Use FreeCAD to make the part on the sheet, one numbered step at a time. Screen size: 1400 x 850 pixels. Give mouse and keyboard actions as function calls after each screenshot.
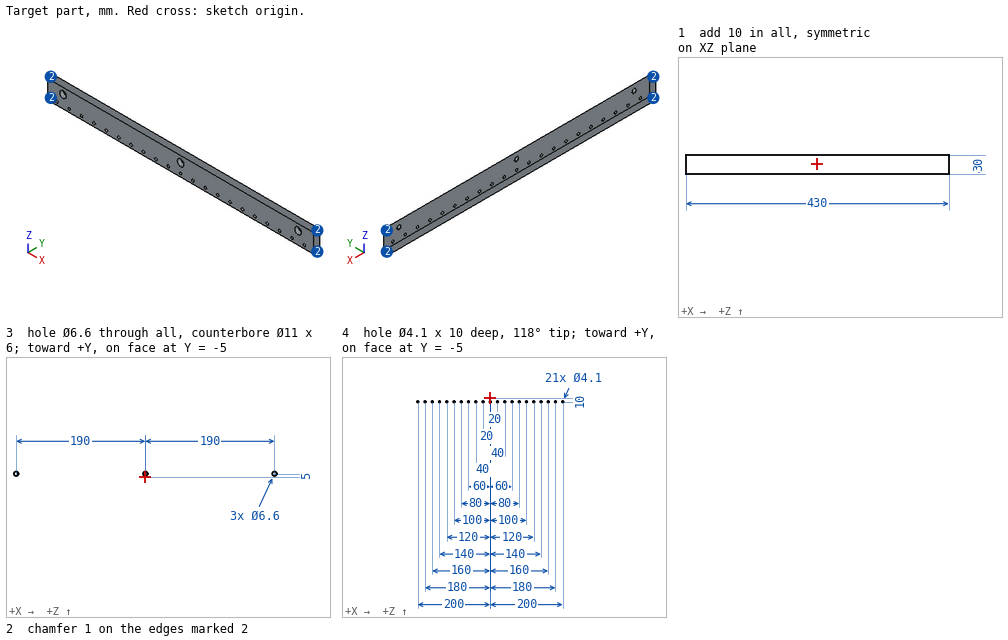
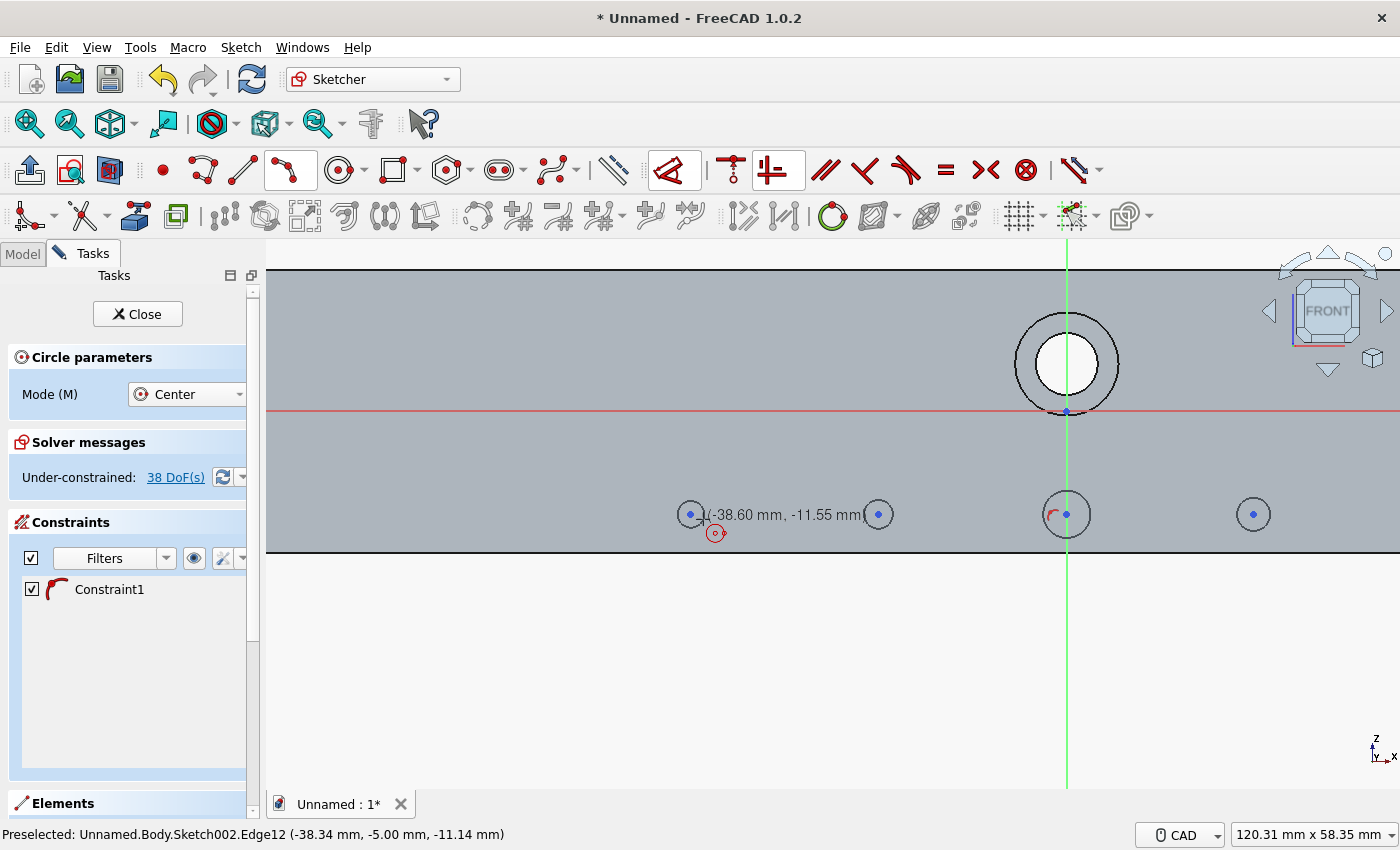
scroll(705, 523, down, 9)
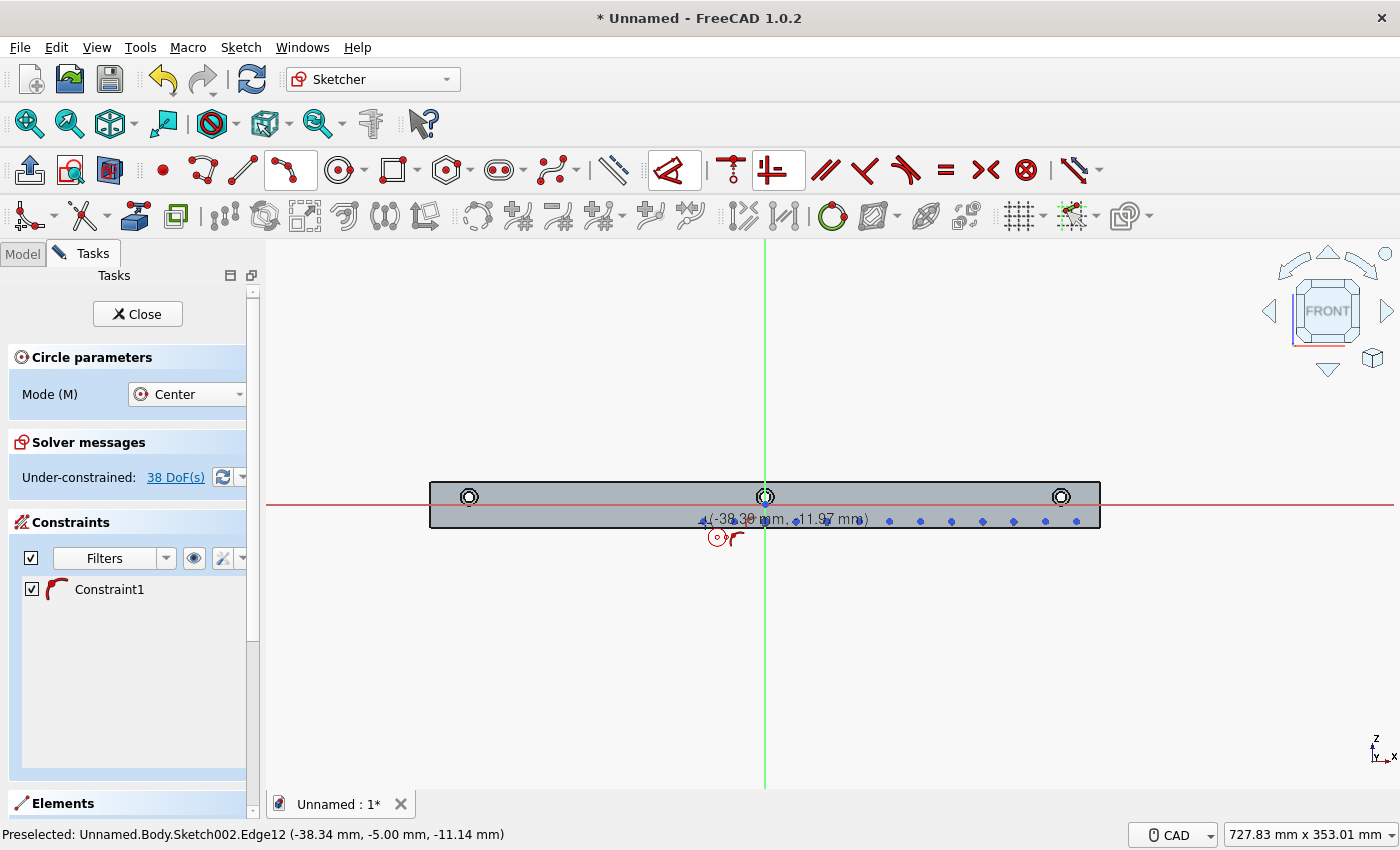
click(672, 521)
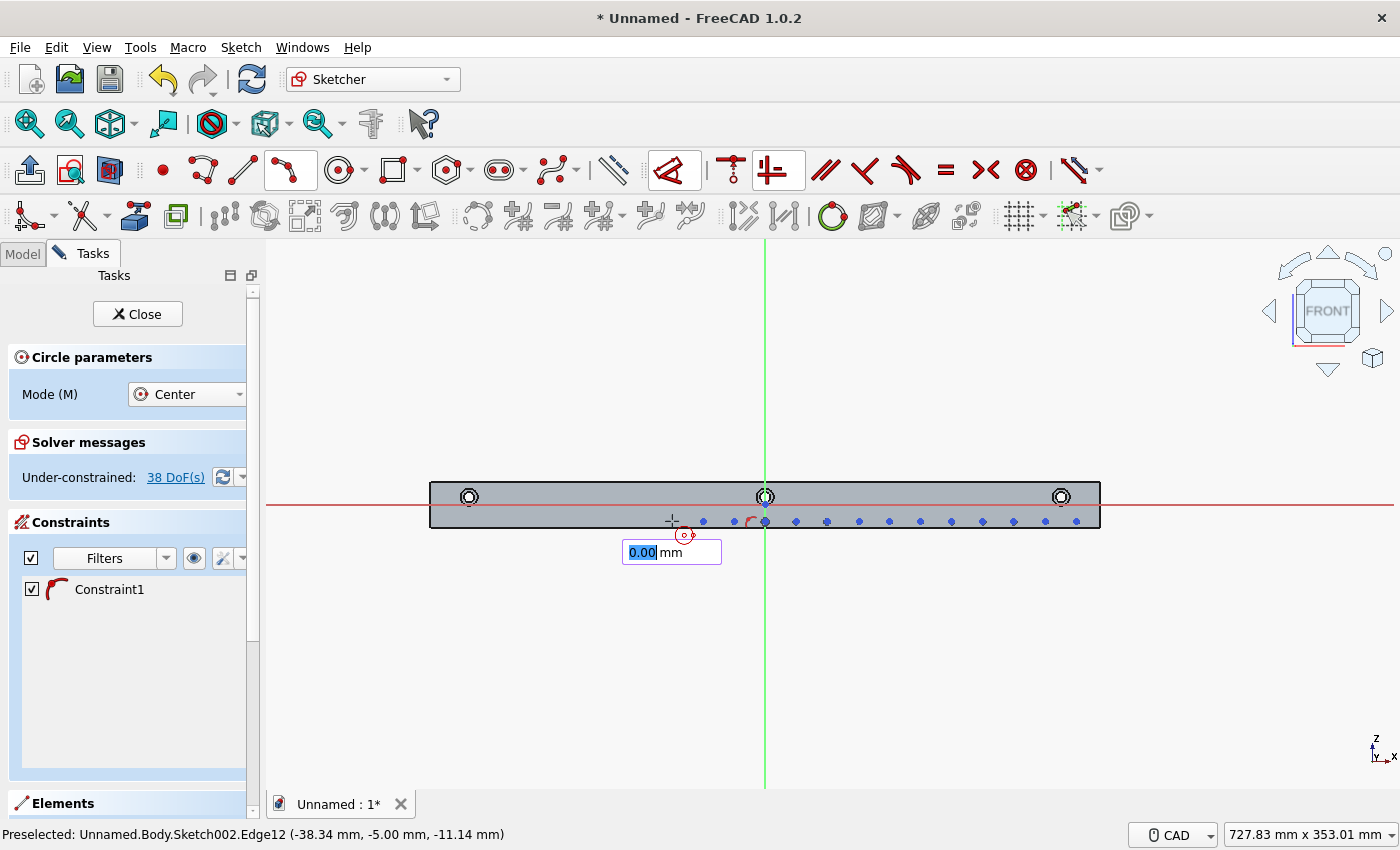
scroll(674, 523, up, 9)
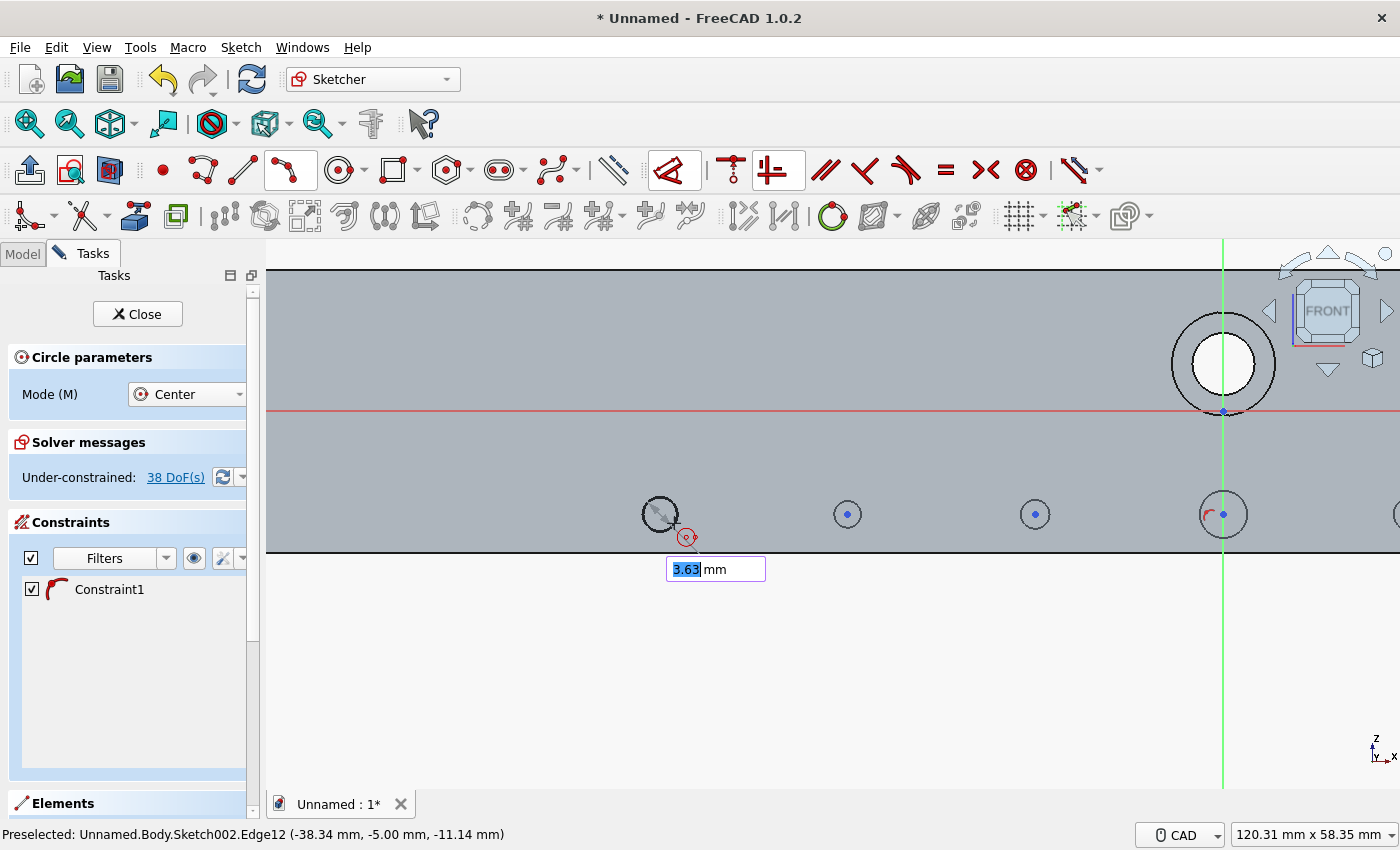
click(672, 519)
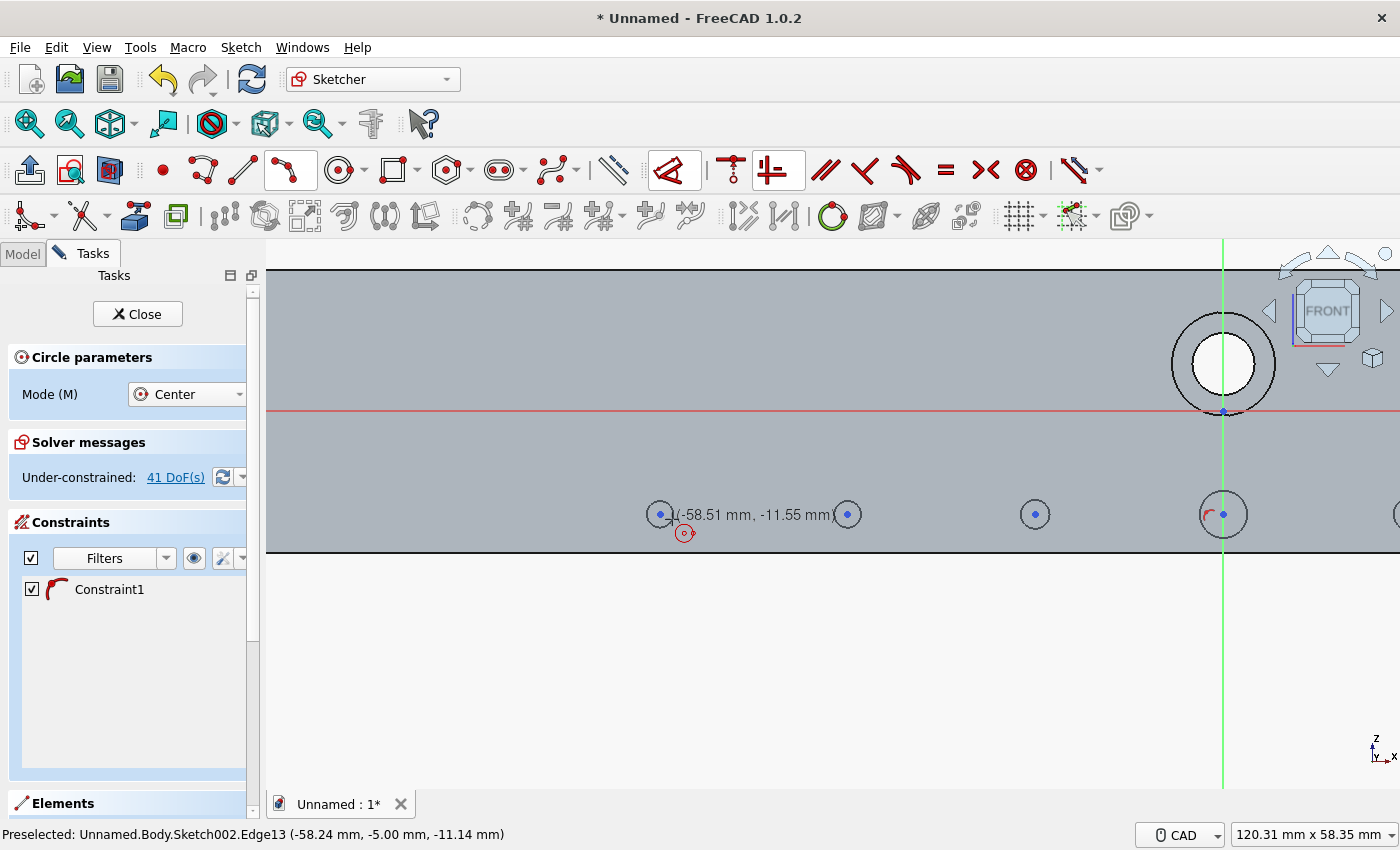
scroll(674, 523, down, 9)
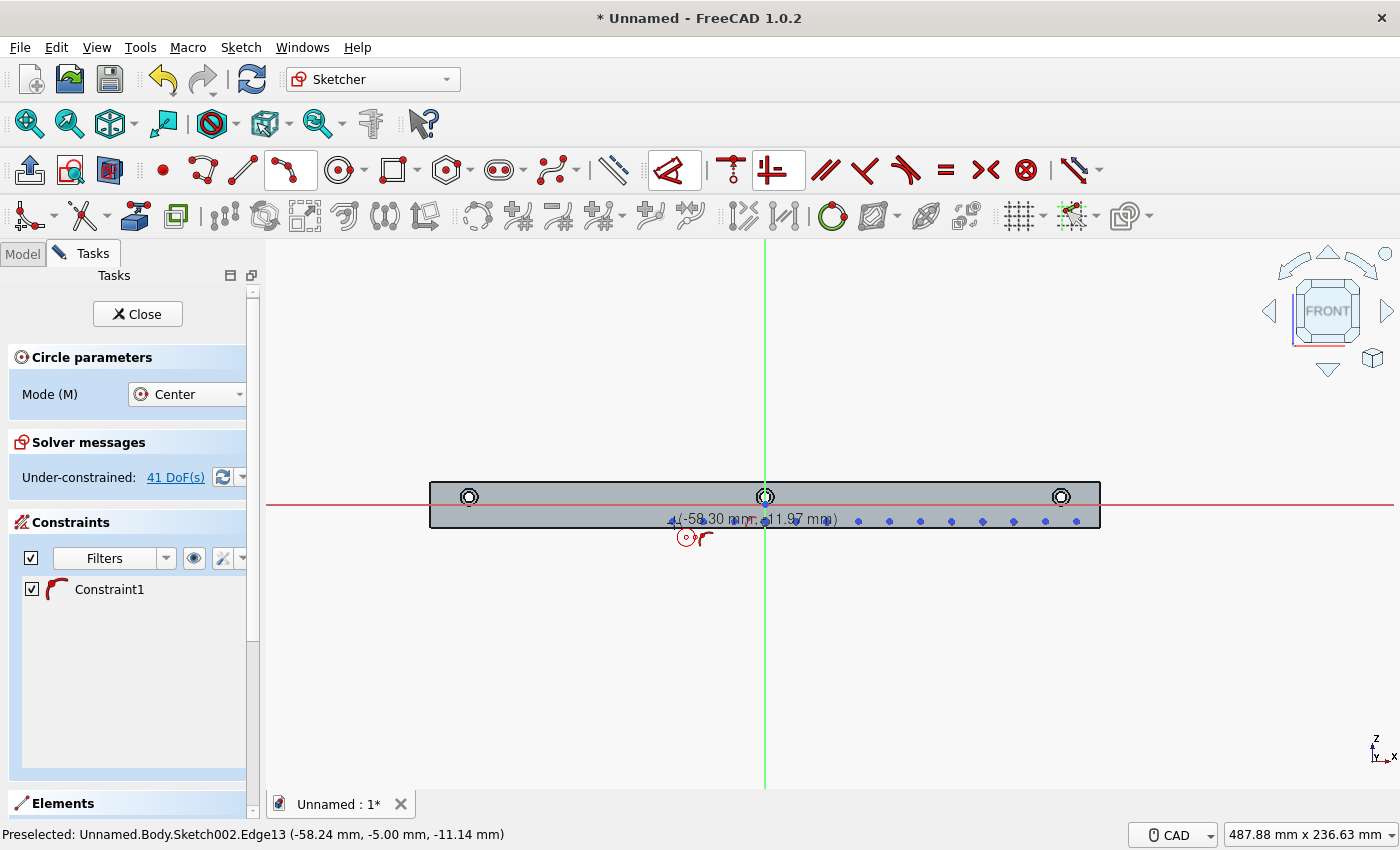
click(640, 521)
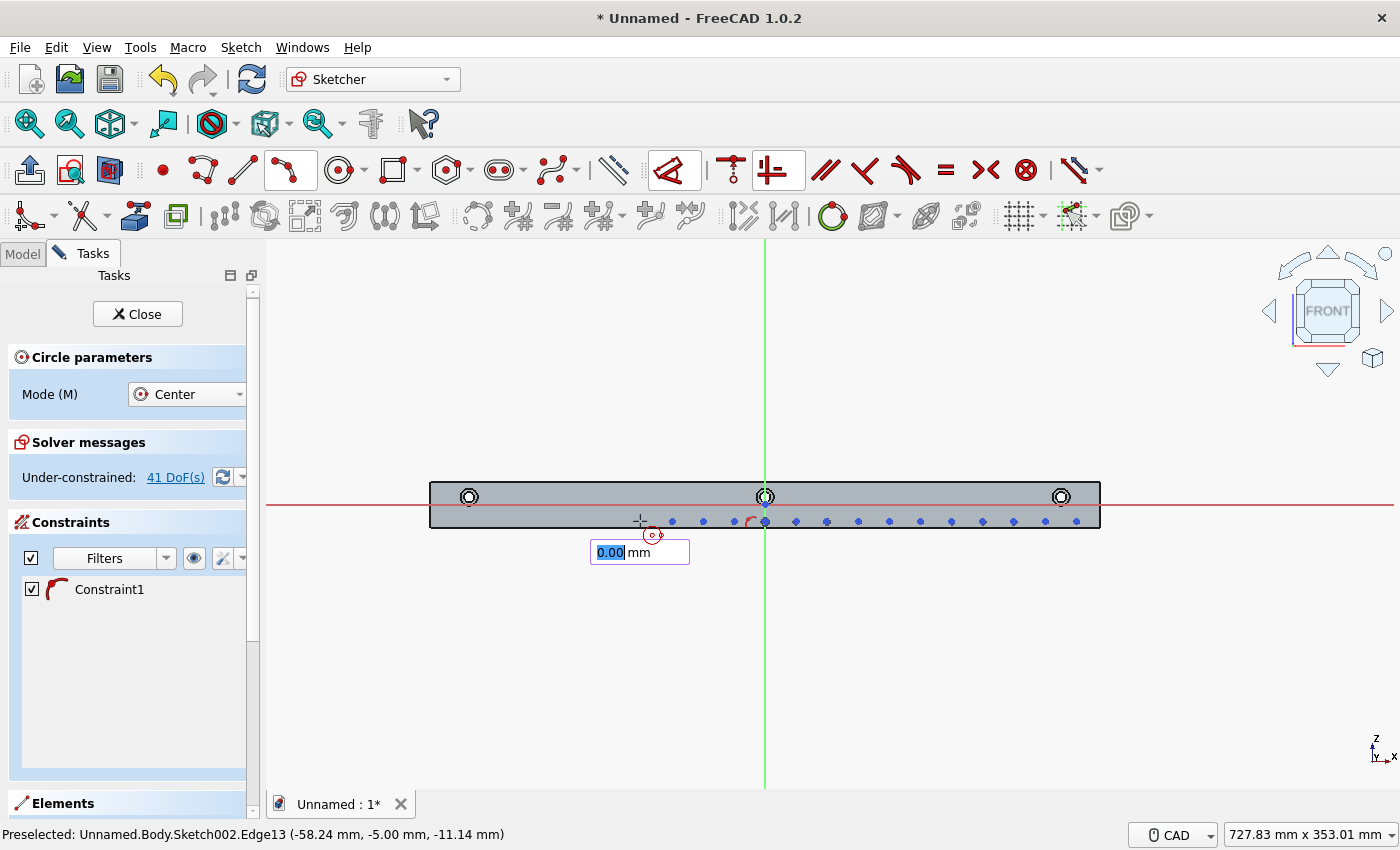
scroll(643, 523, up, 9)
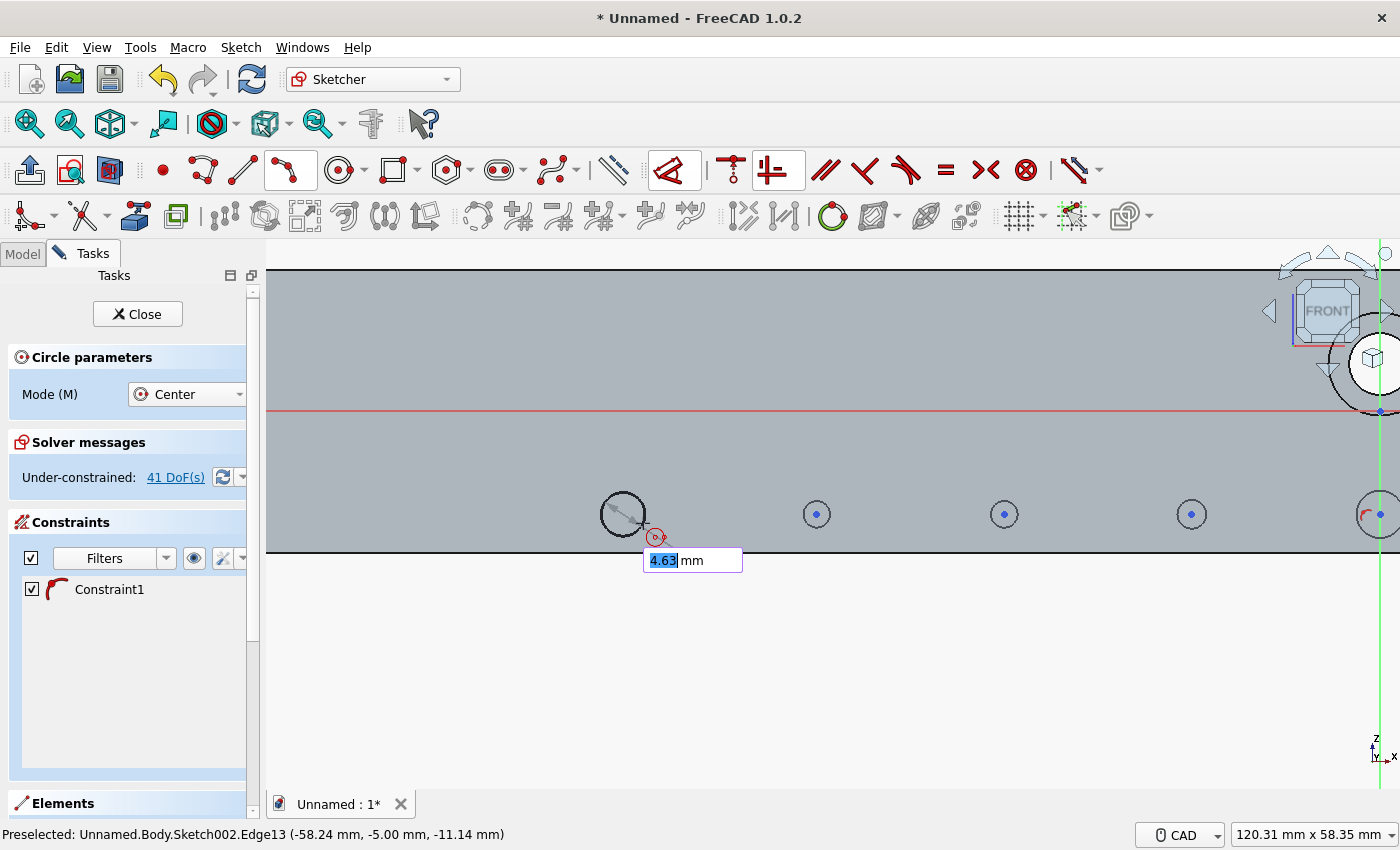
click(640, 519)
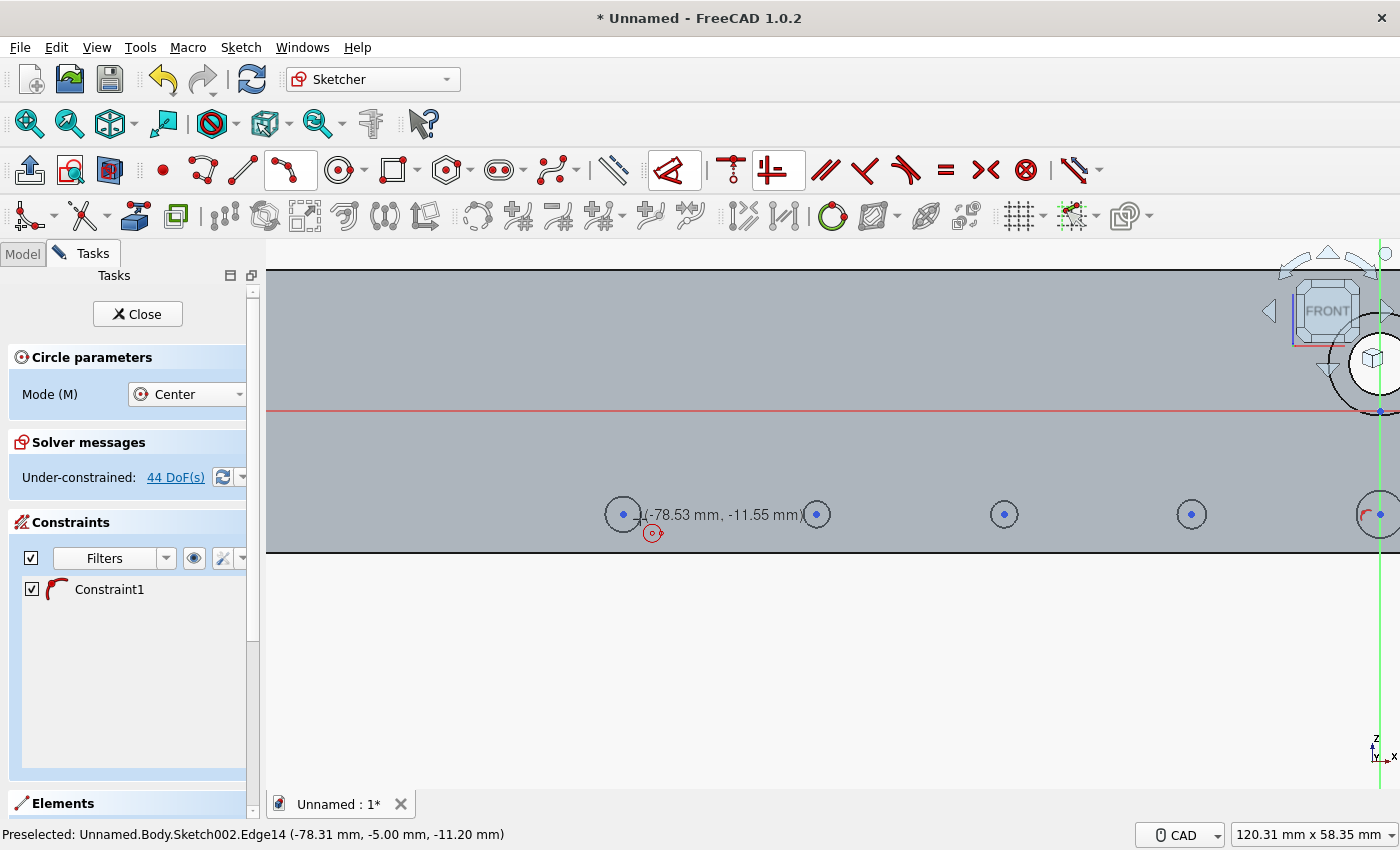
scroll(643, 523, down, 9)